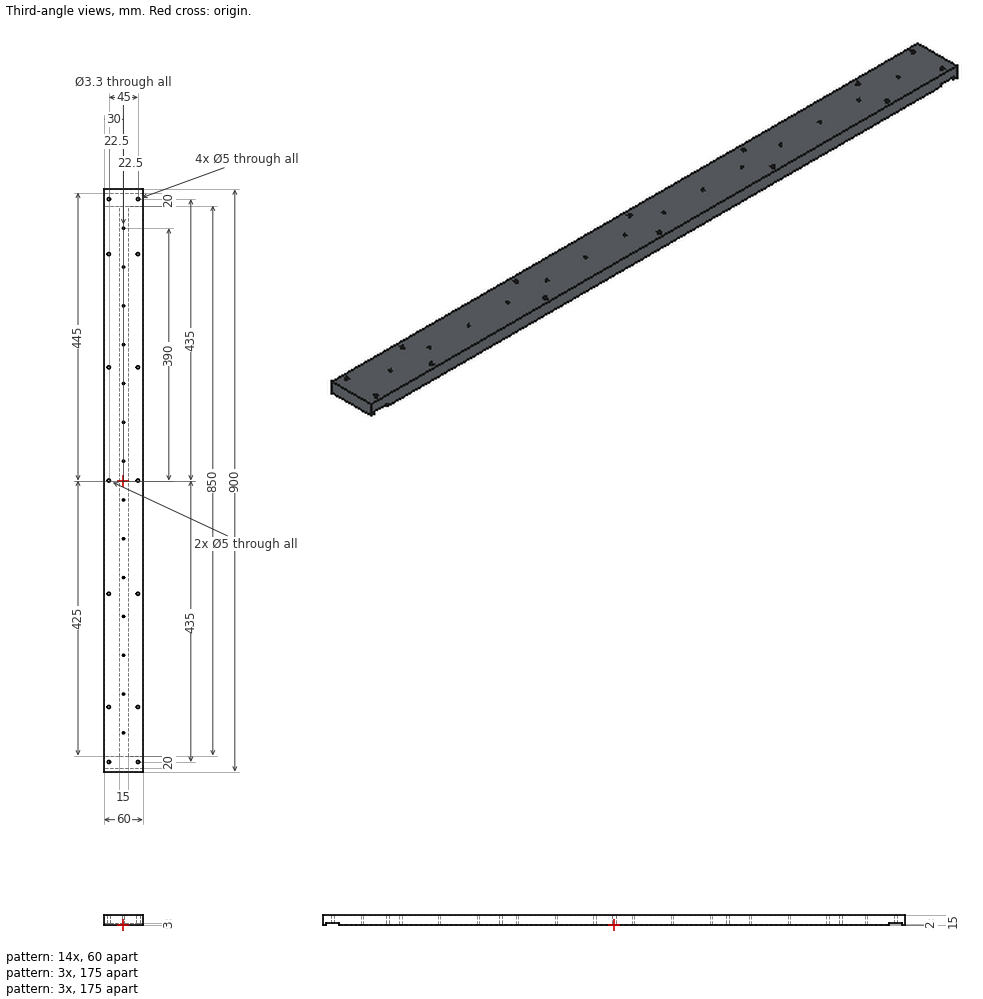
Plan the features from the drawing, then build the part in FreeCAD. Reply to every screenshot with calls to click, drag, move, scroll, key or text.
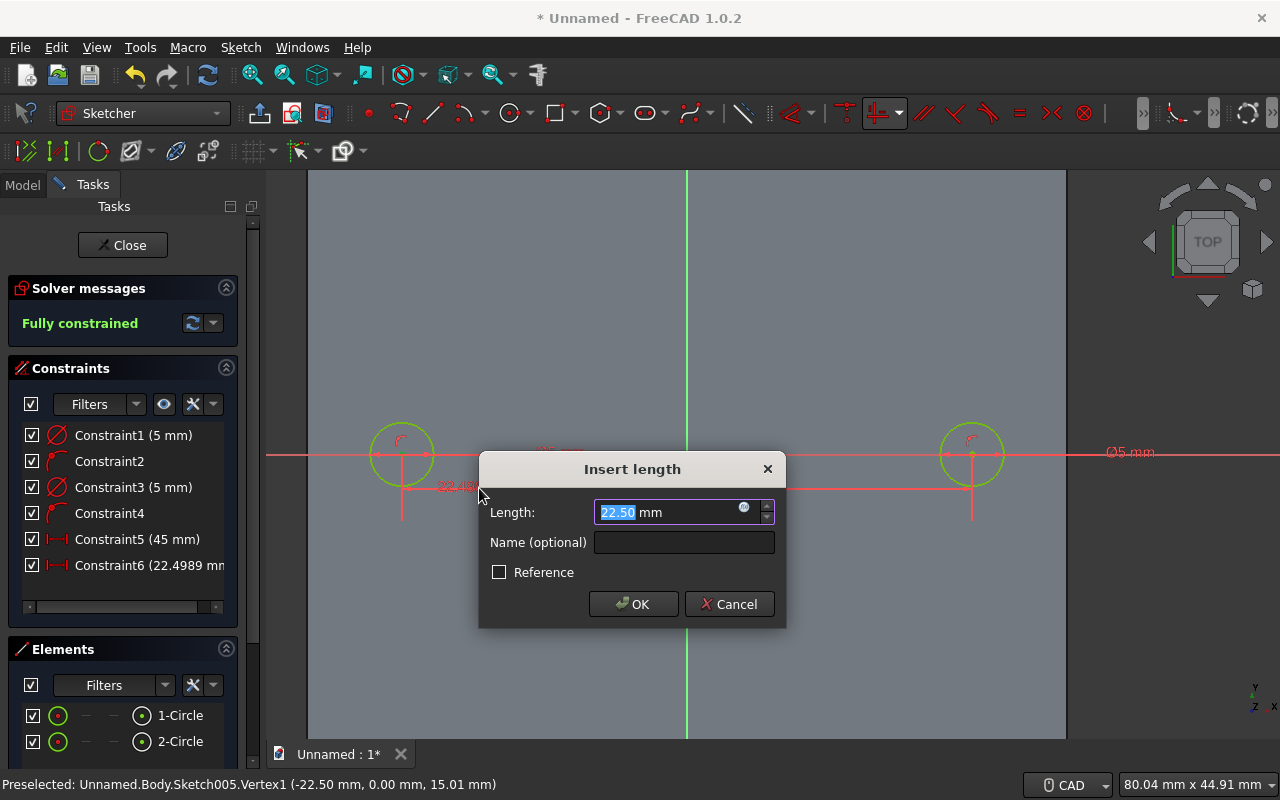
text(22.5)
key(Return)
key(Escape)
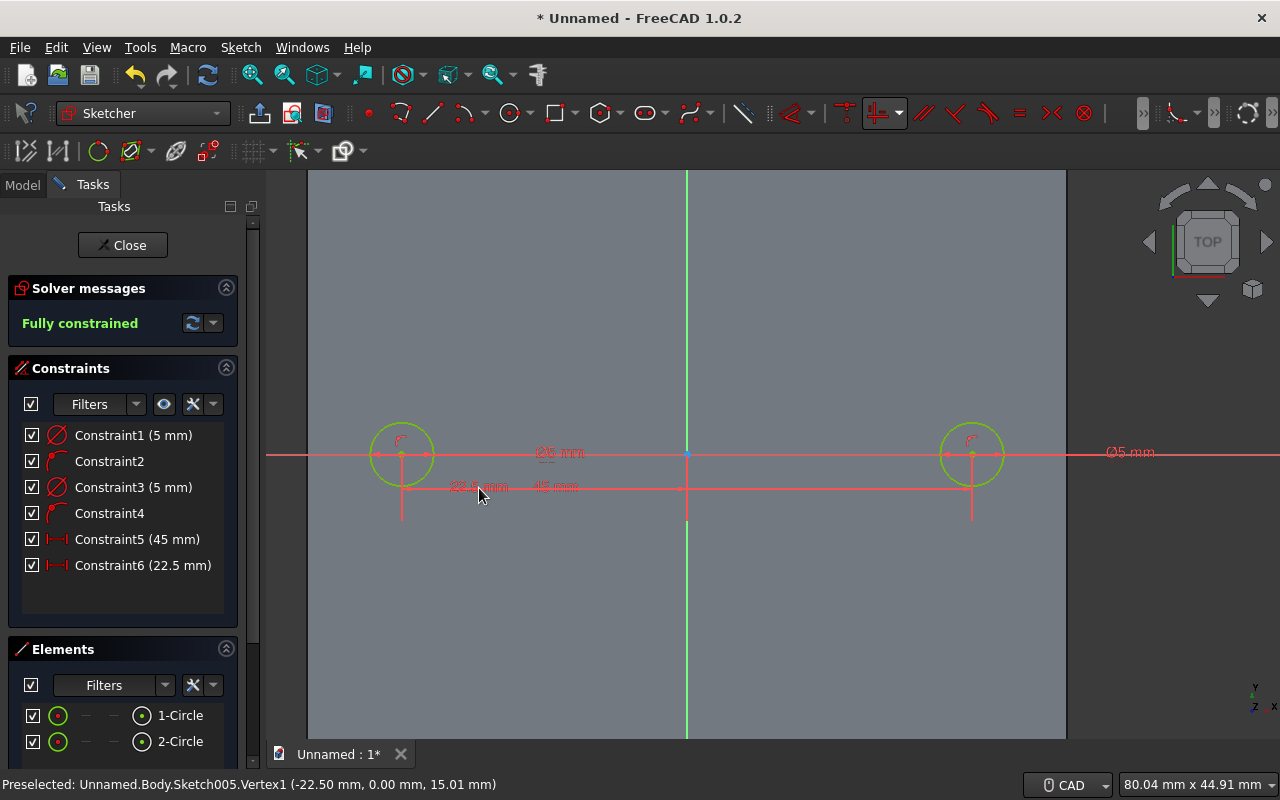
click(123, 245)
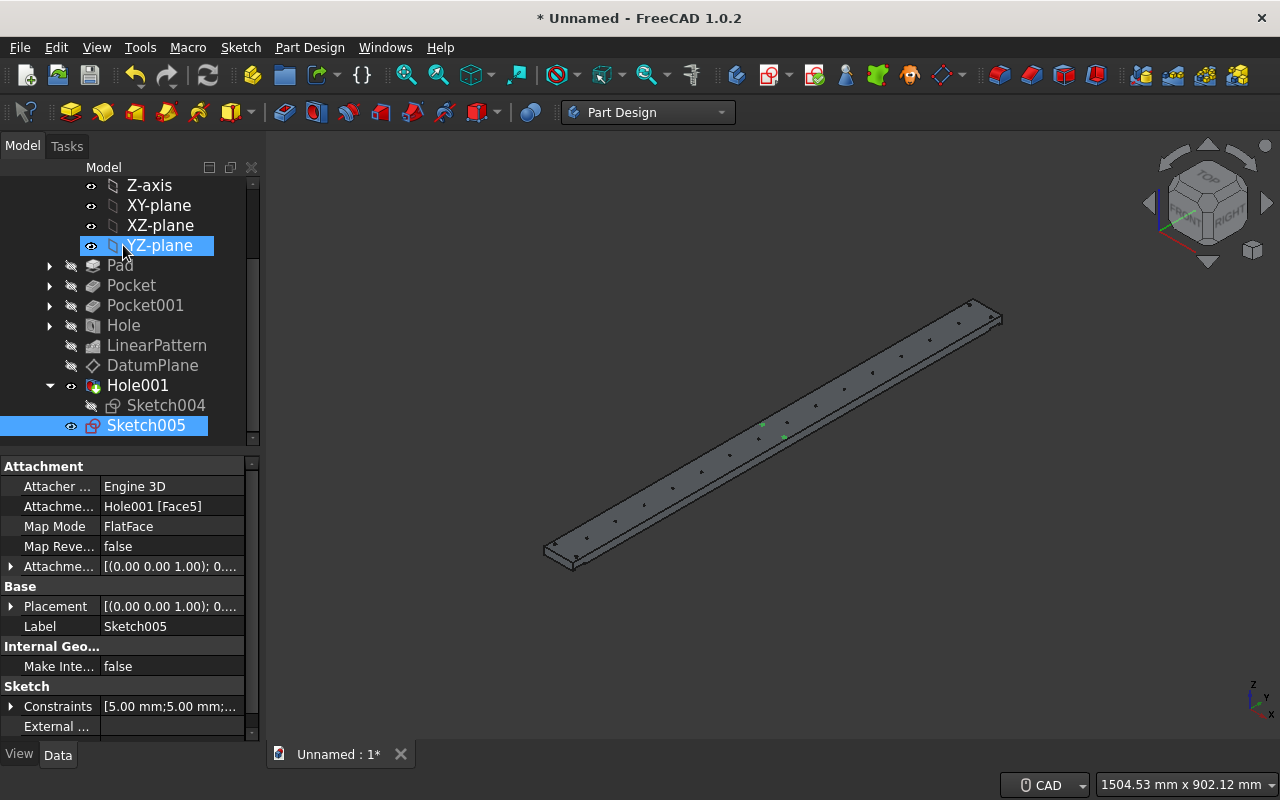
click(318, 112)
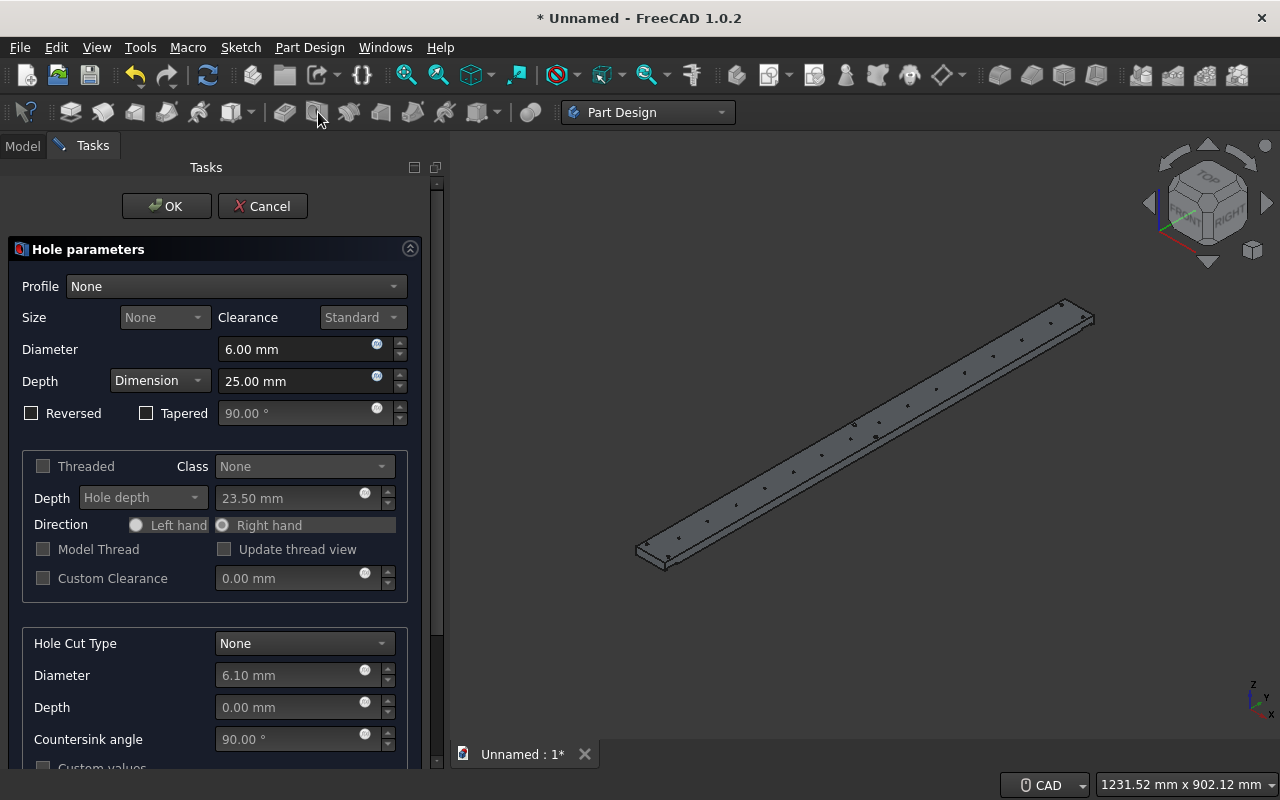
triple_click(305, 349)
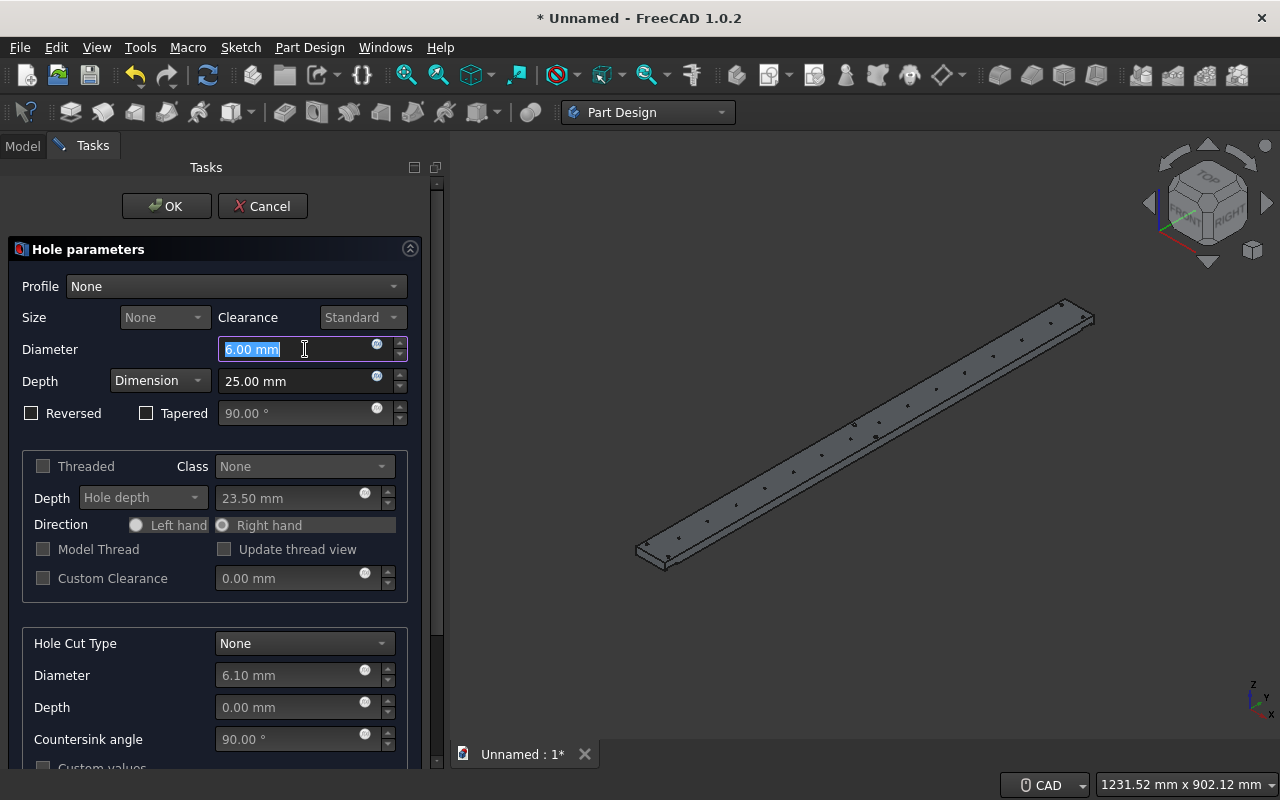
text(5)
key(Tab)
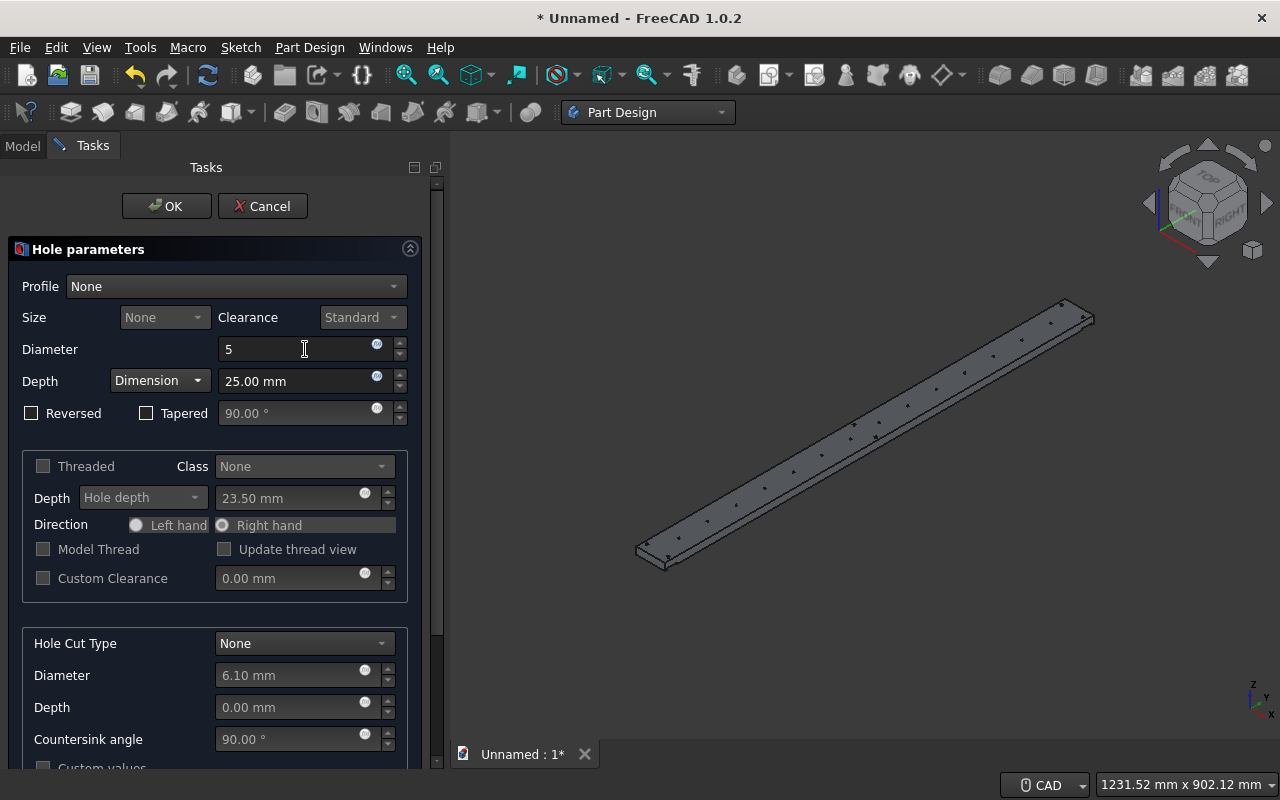
click(161, 380)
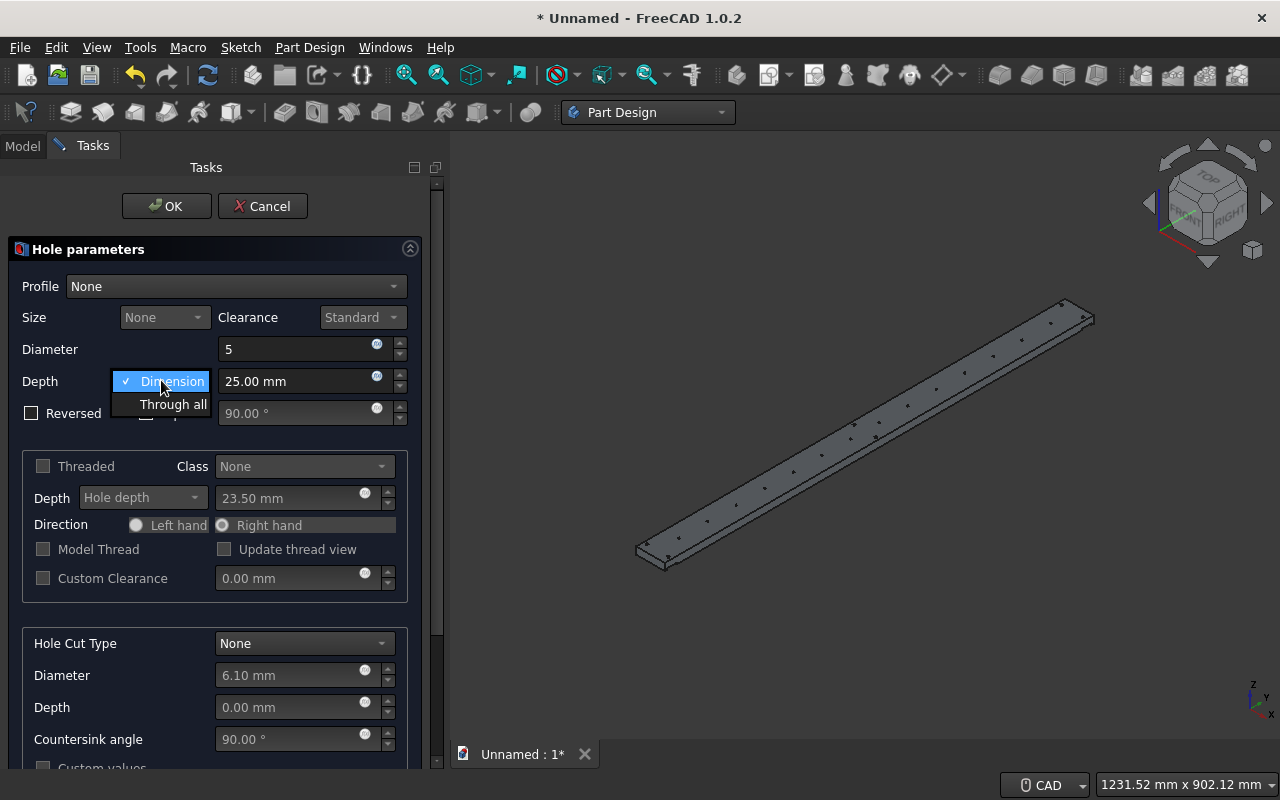
click(160, 404)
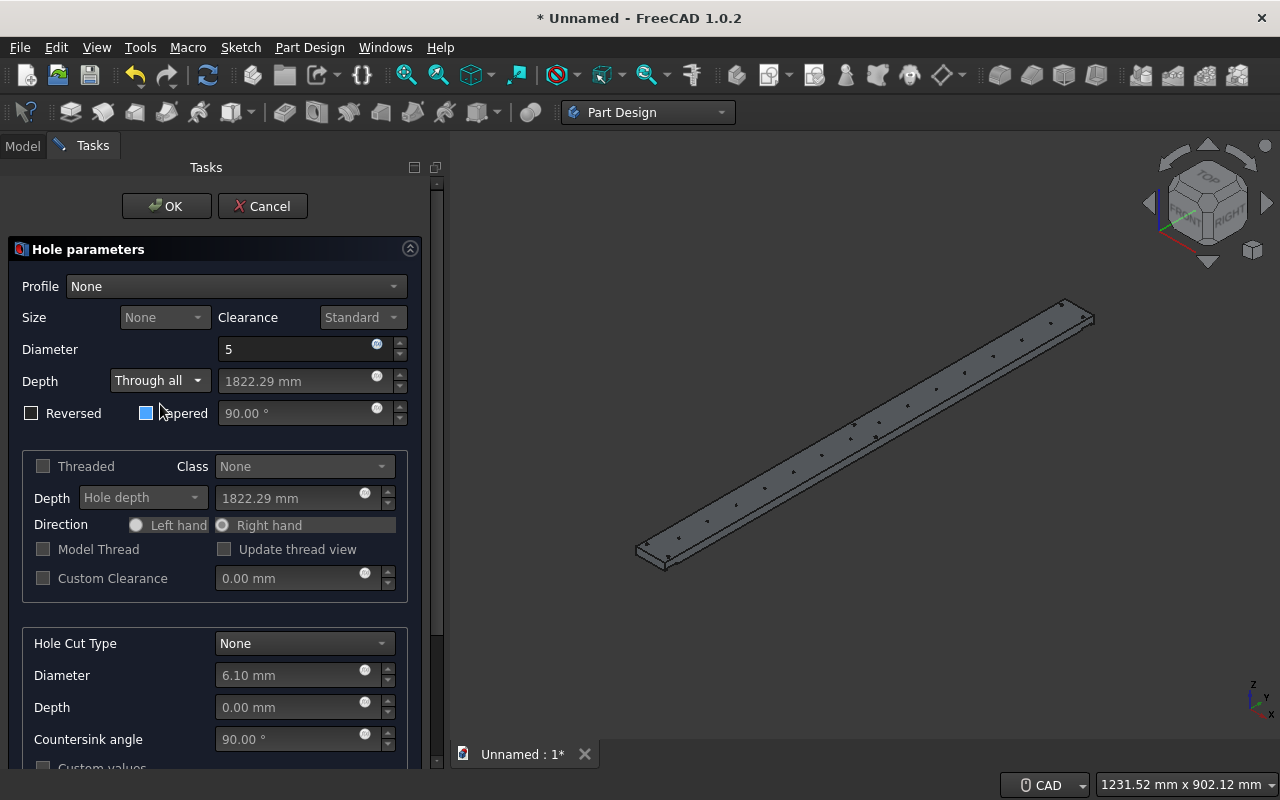
click(167, 206)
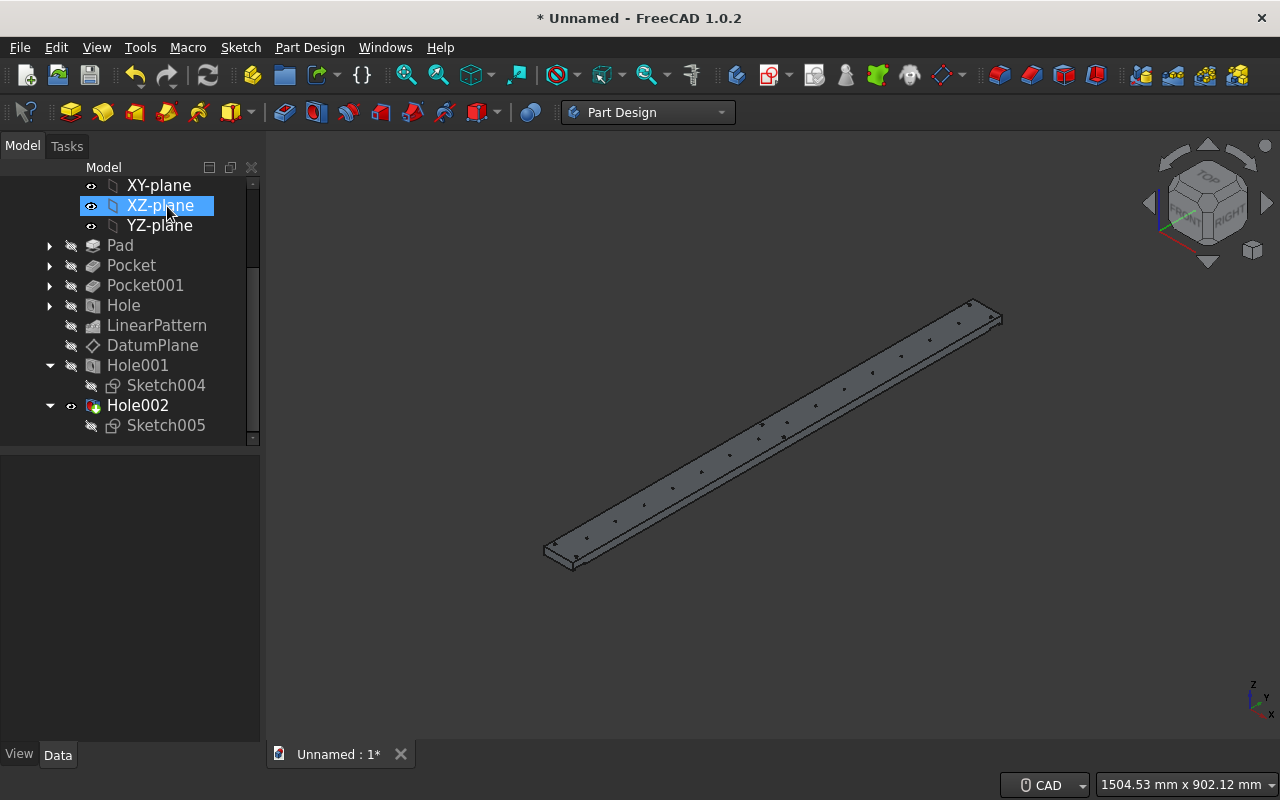
click(116, 406)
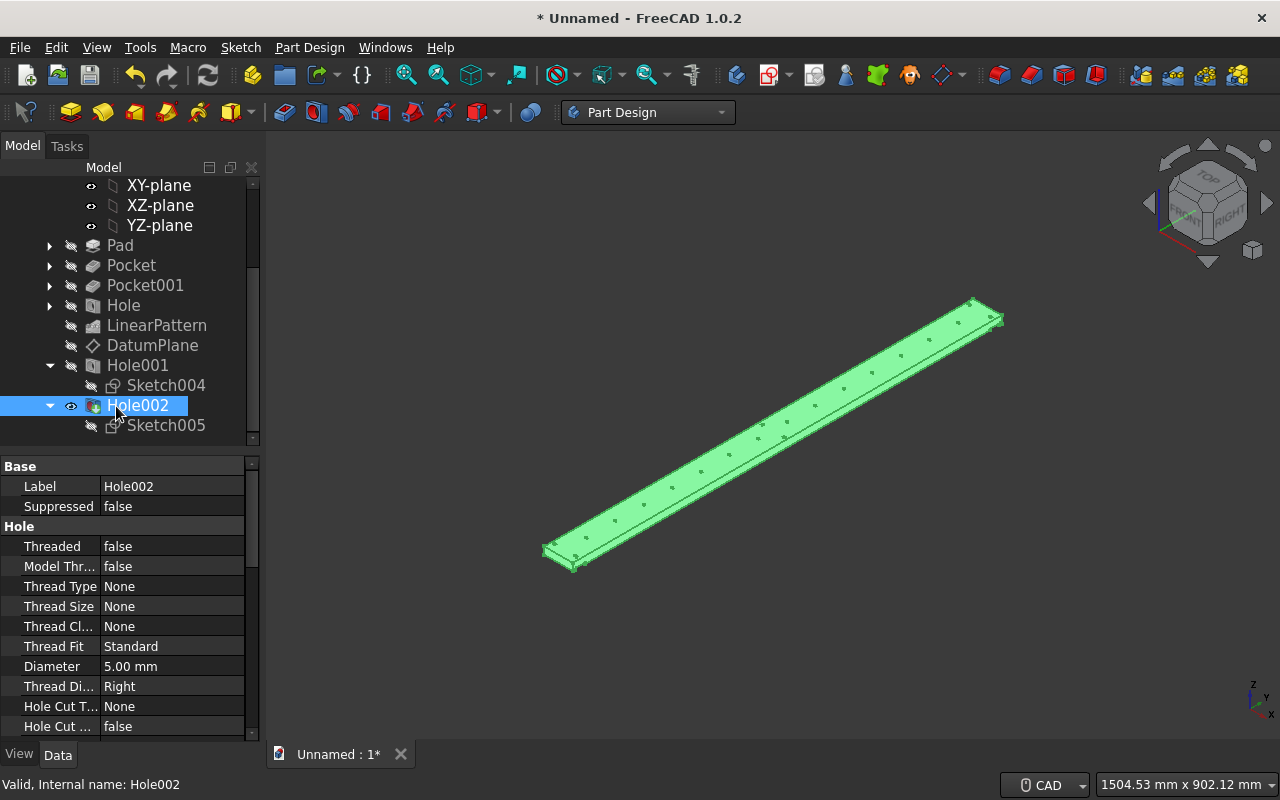
click(1174, 76)